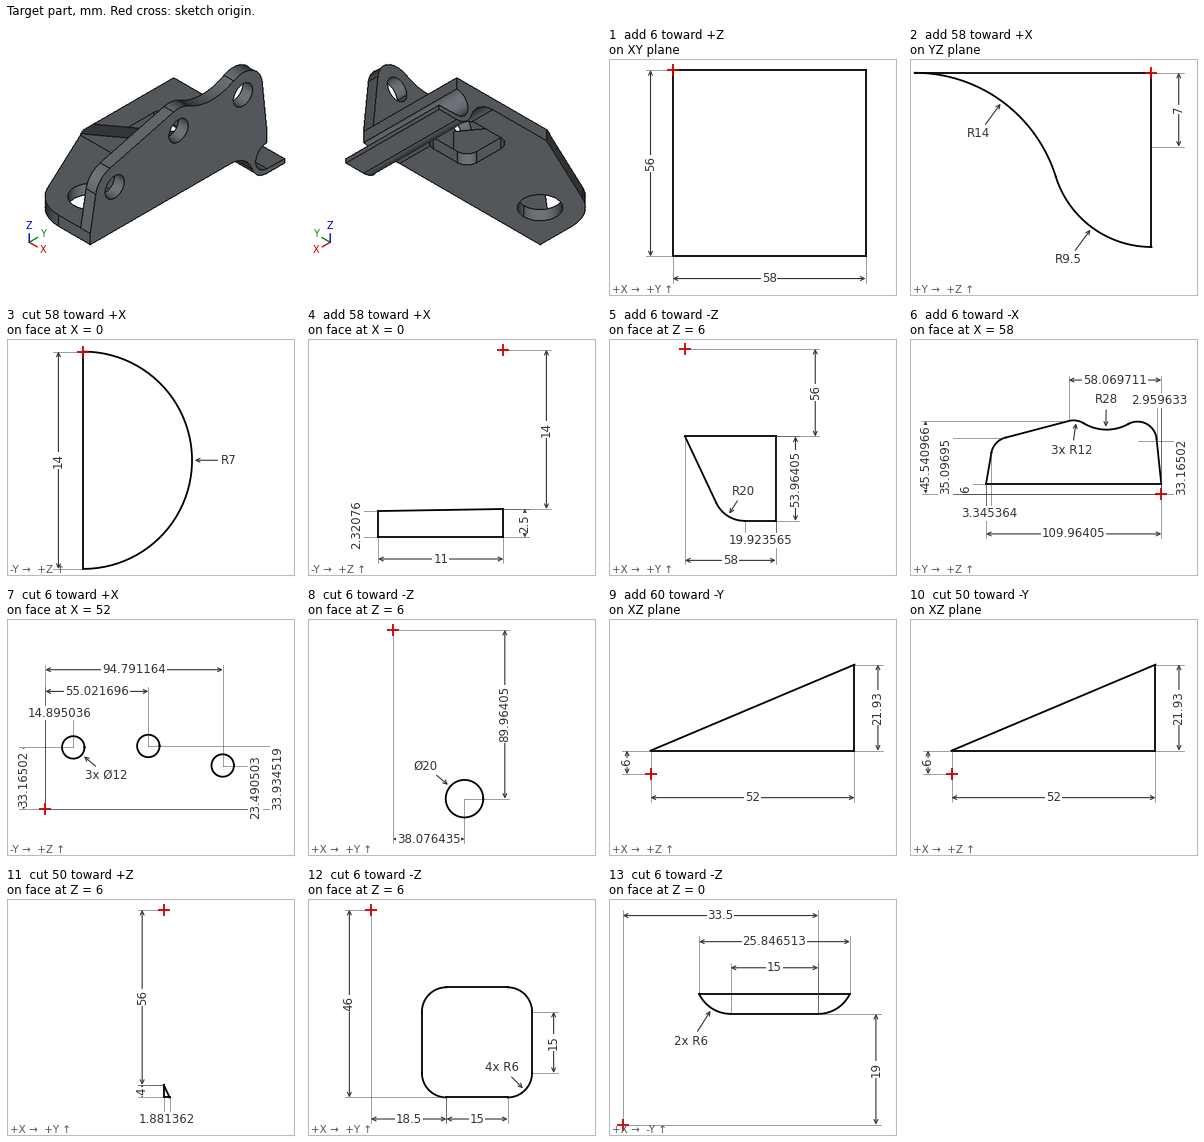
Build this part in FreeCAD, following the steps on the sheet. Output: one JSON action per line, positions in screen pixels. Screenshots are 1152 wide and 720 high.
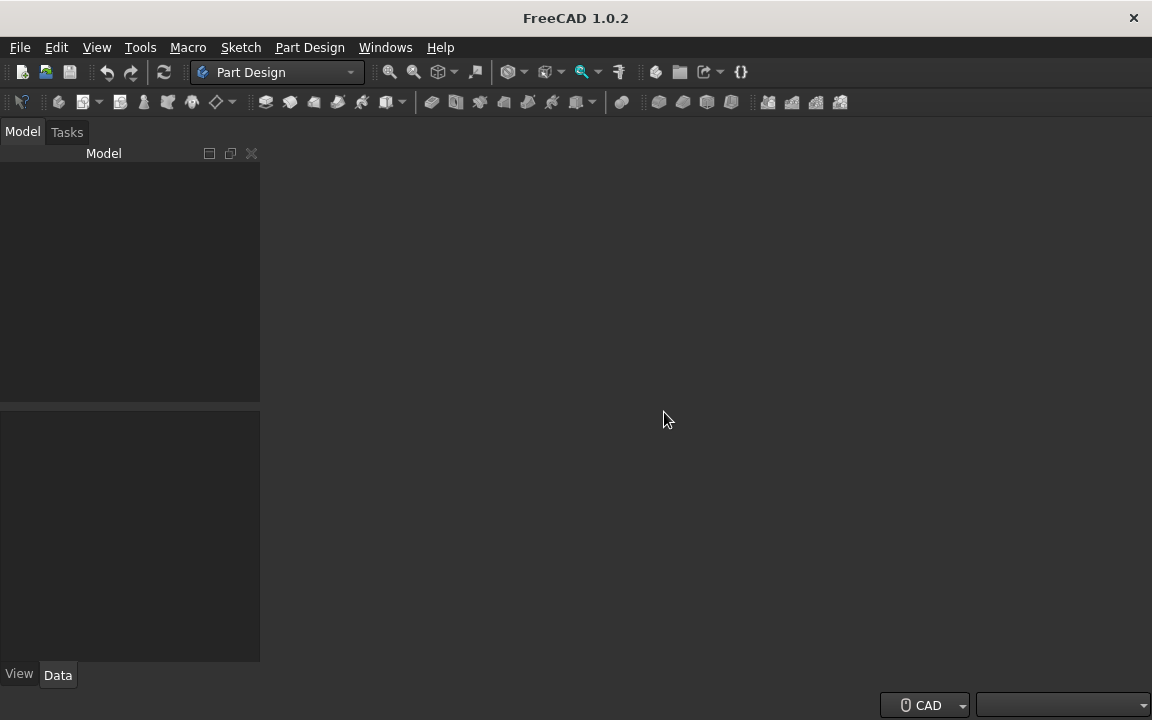
{"action": "left_click", "coordinate": [22, 72]}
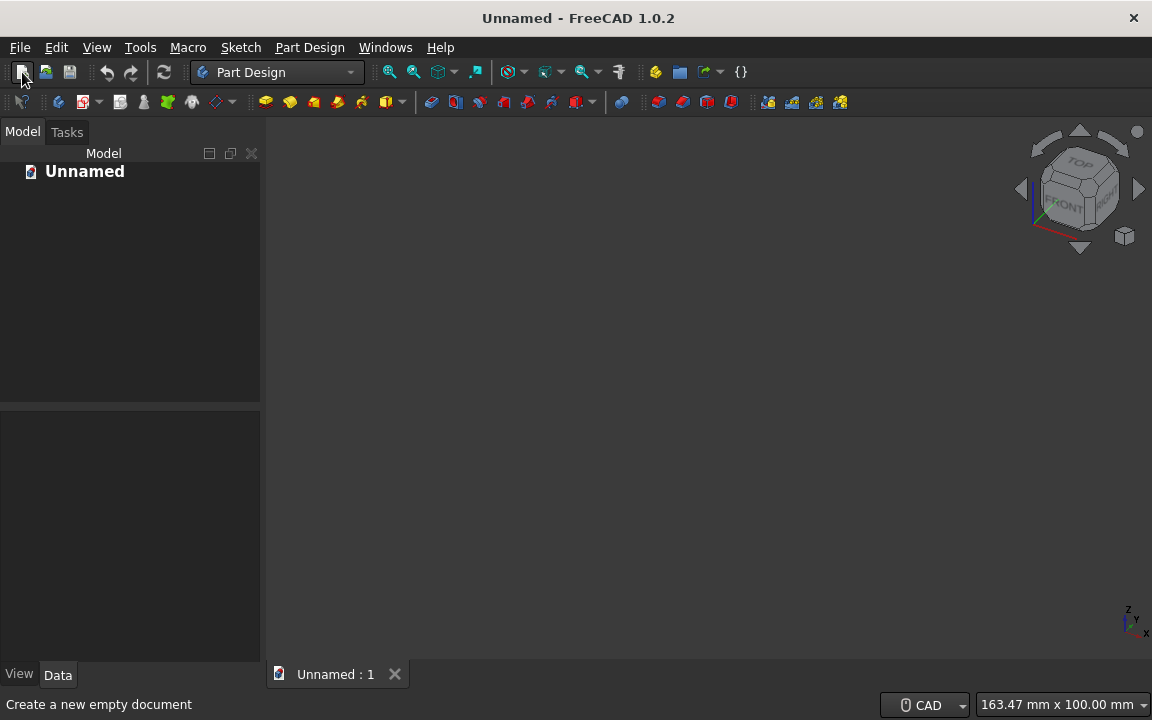
{"action": "left_click", "coordinate": [84, 102]}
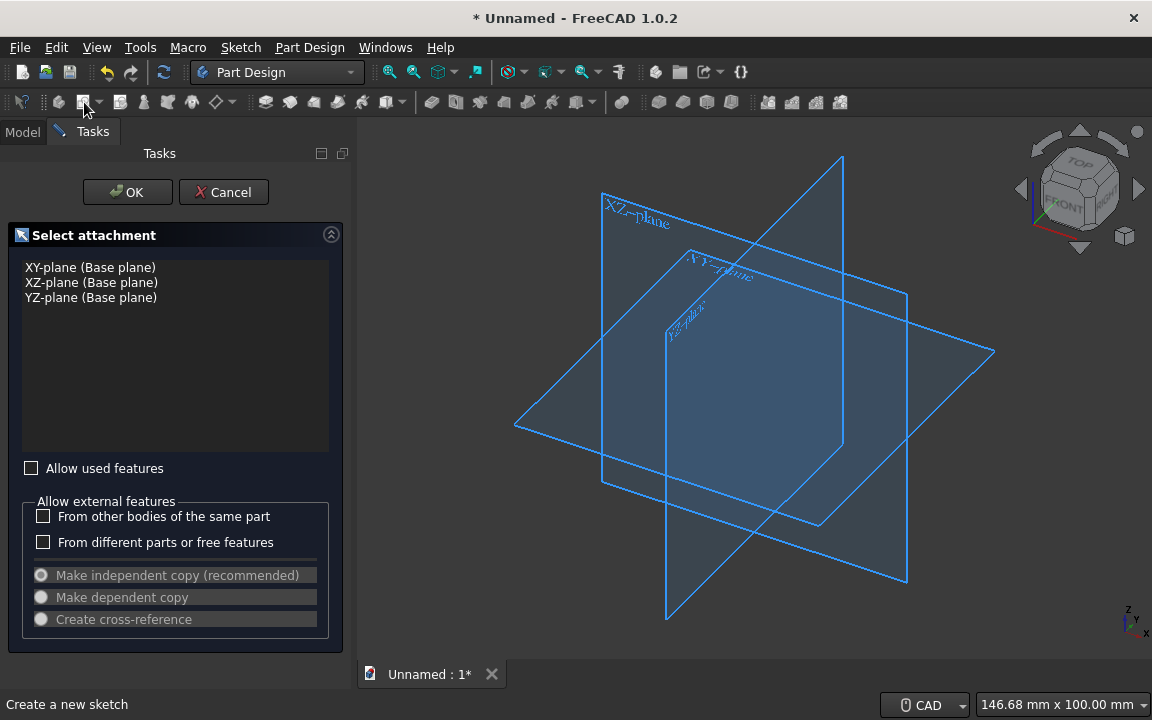
{"action": "left_click", "coordinate": [82, 268]}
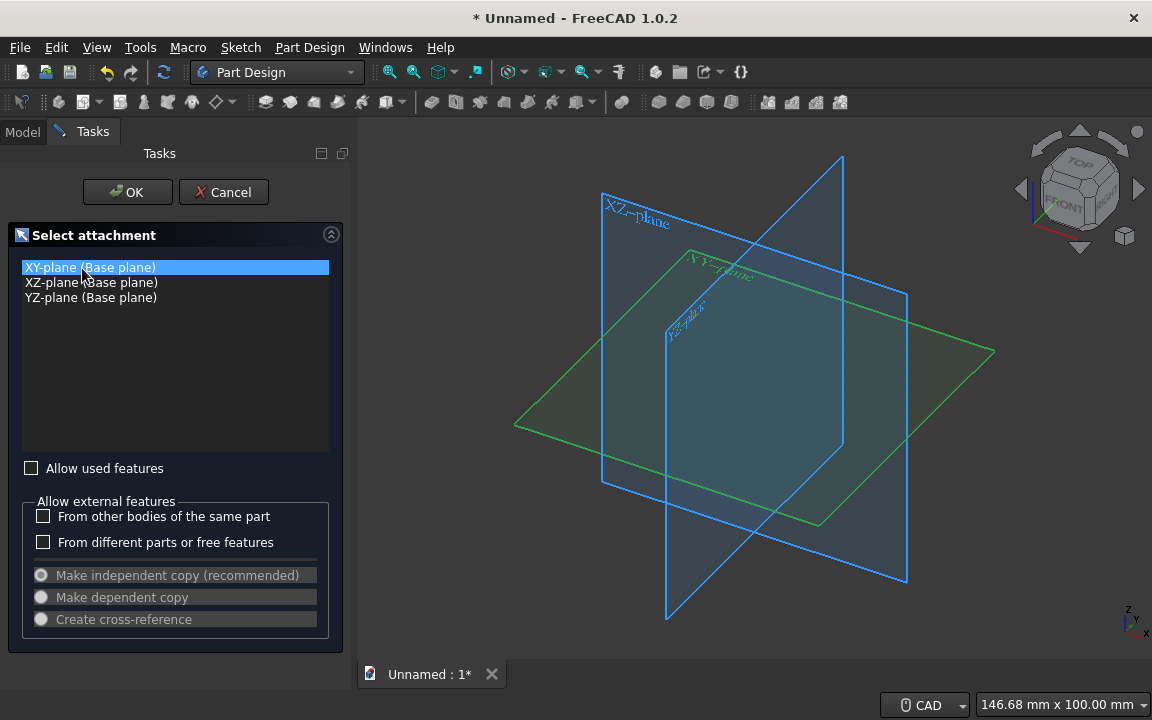
{"action": "left_click", "coordinate": [128, 192]}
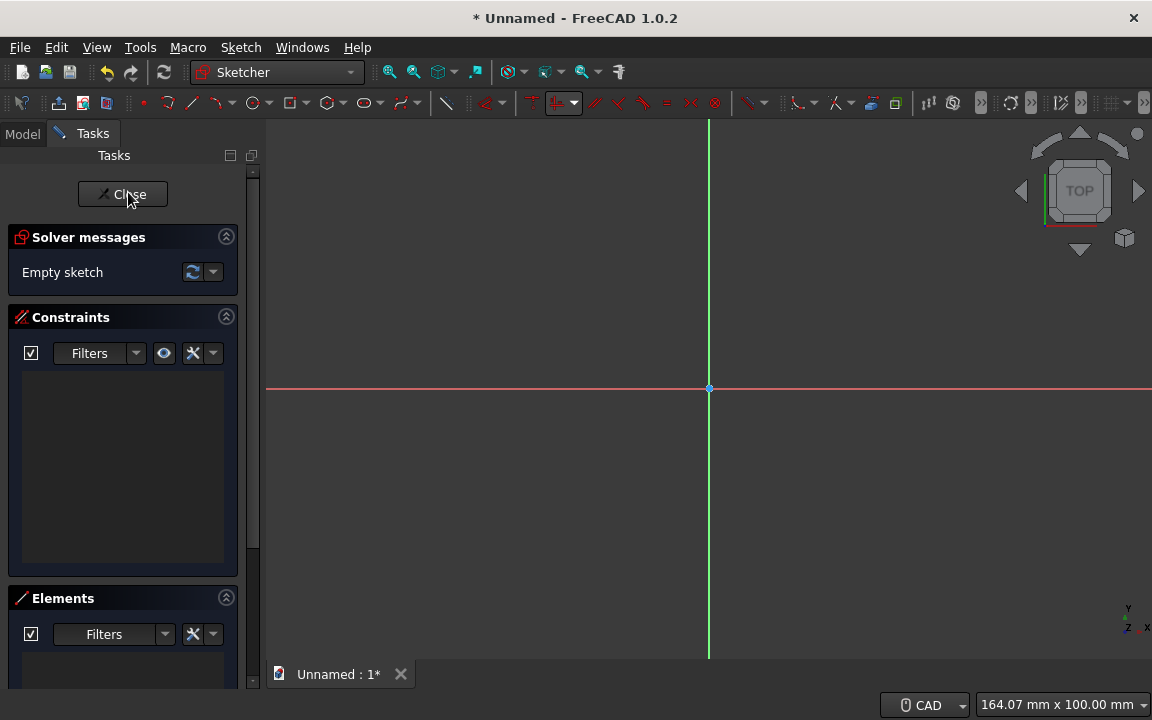
{"action": "scroll", "coordinate": [294, 147], "scroll_direction": "down", "scroll_amount": 1}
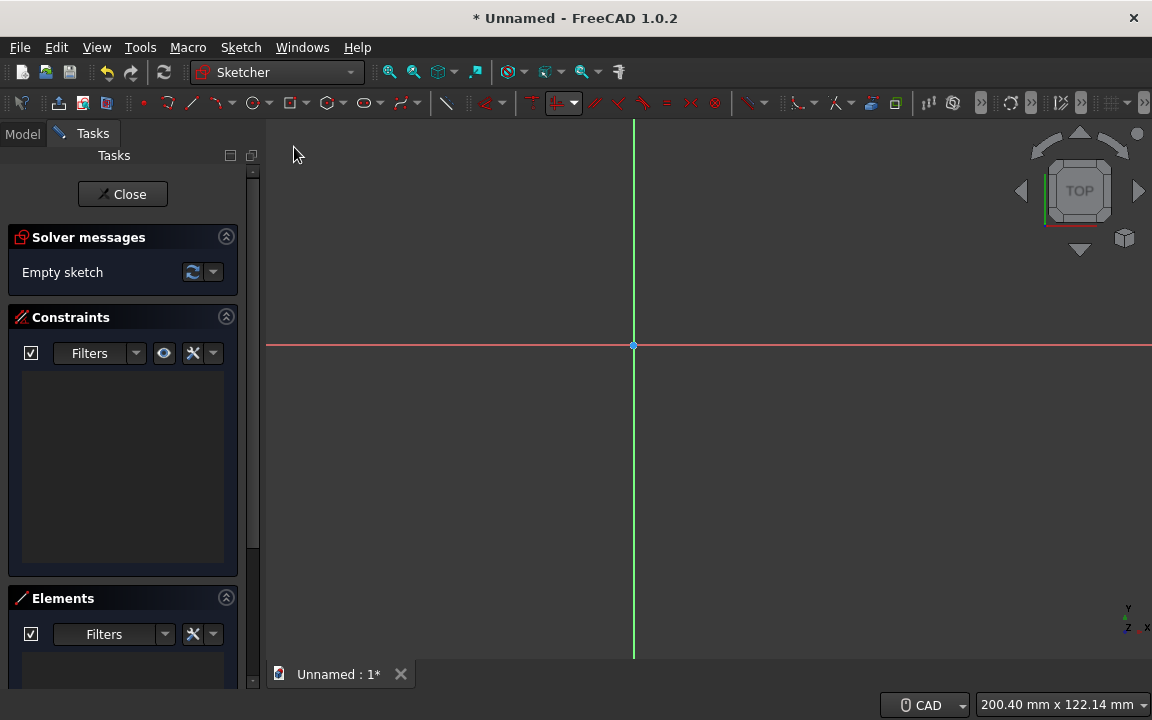
{"action": "scroll", "coordinate": [987, 631], "scroll_direction": "up", "scroll_amount": 2}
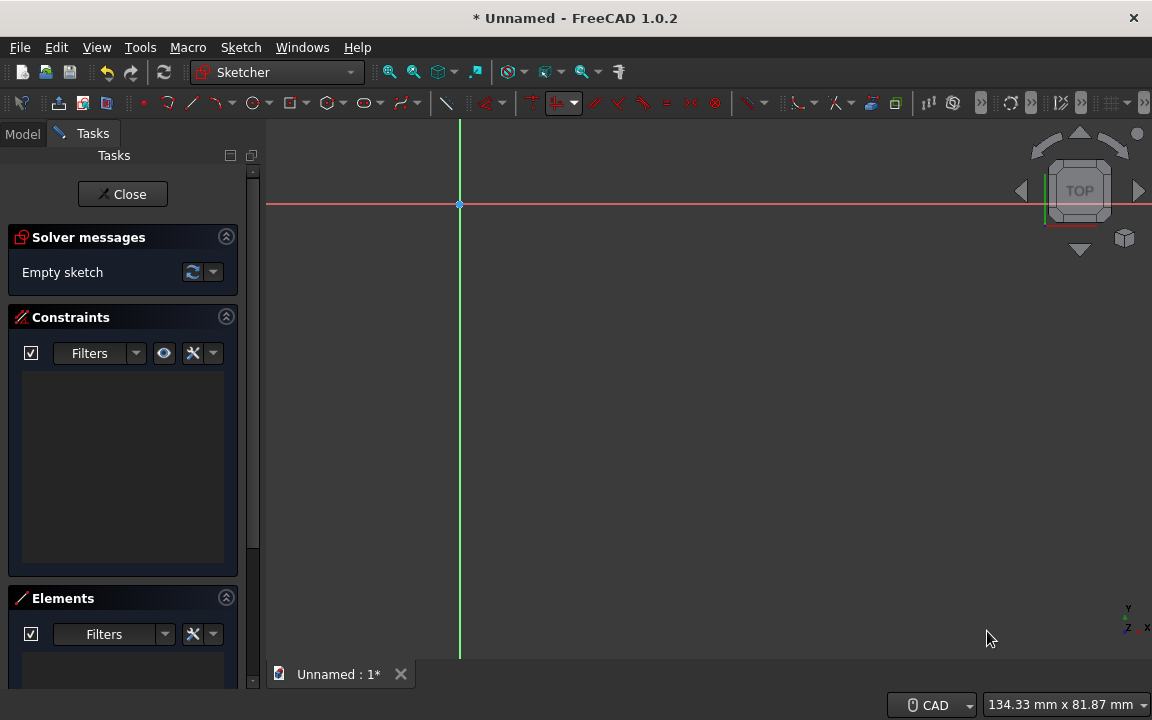
{"action": "key", "text": "g r"}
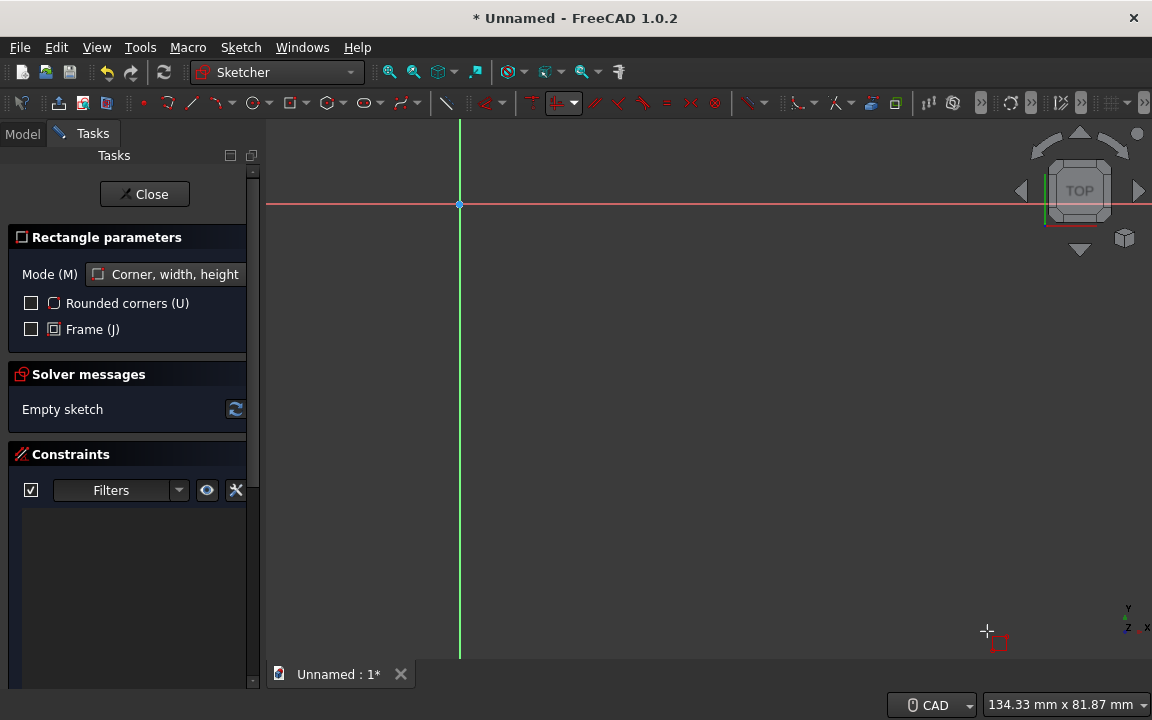
{"action": "left_click", "coordinate": [460, 204]}
{"action": "left_click", "coordinate": [842, 573]}
{"action": "key", "text": "Escape"}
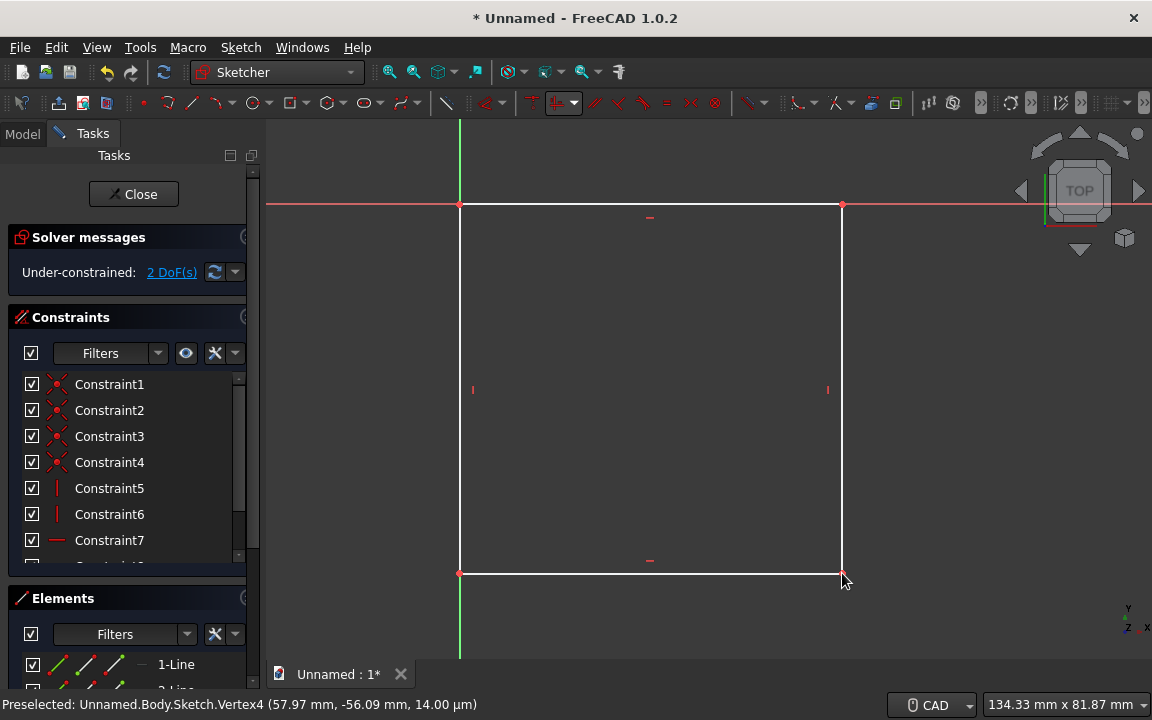
{"action": "left_click", "coordinate": [486, 104]}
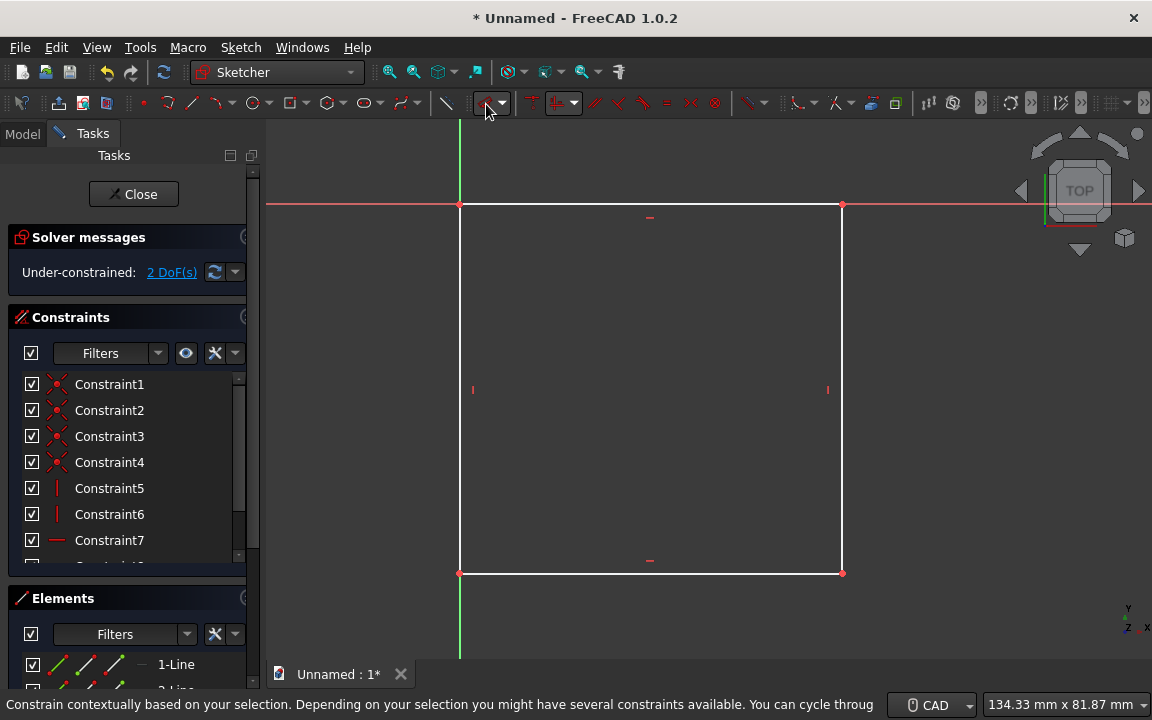
{"action": "left_click", "coordinate": [460, 315]}
{"action": "left_click", "coordinate": [426, 389]}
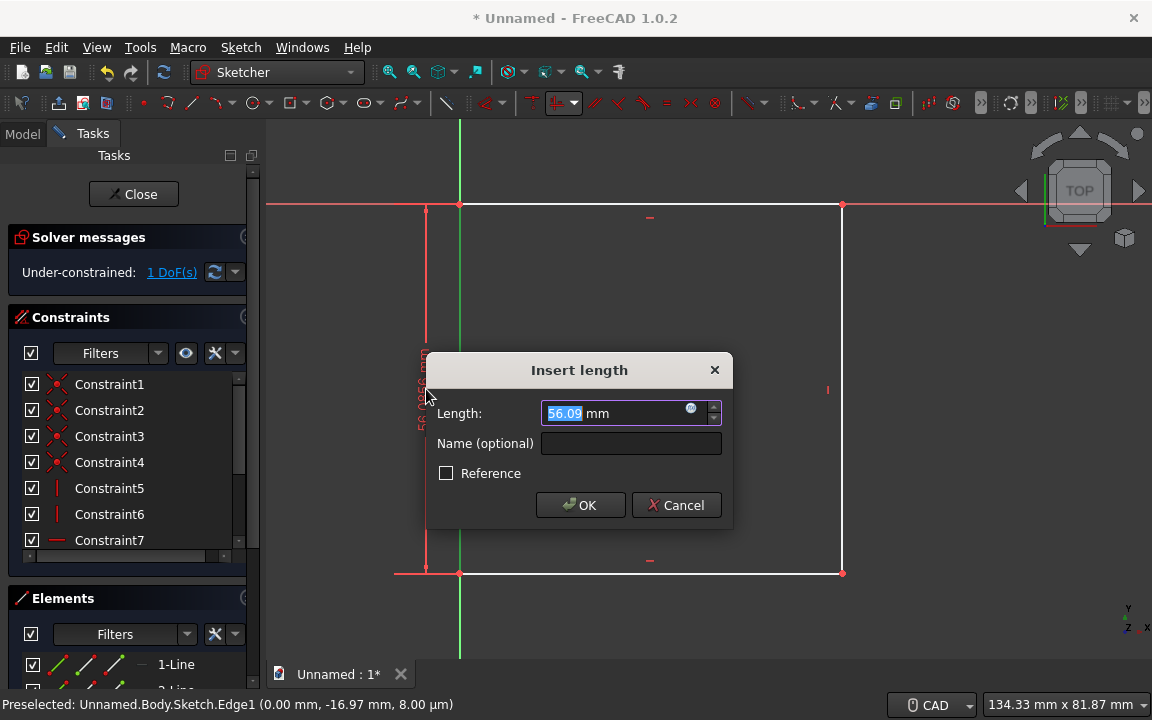
{"action": "type", "text": "56"}
{"action": "key", "text": "Return"}